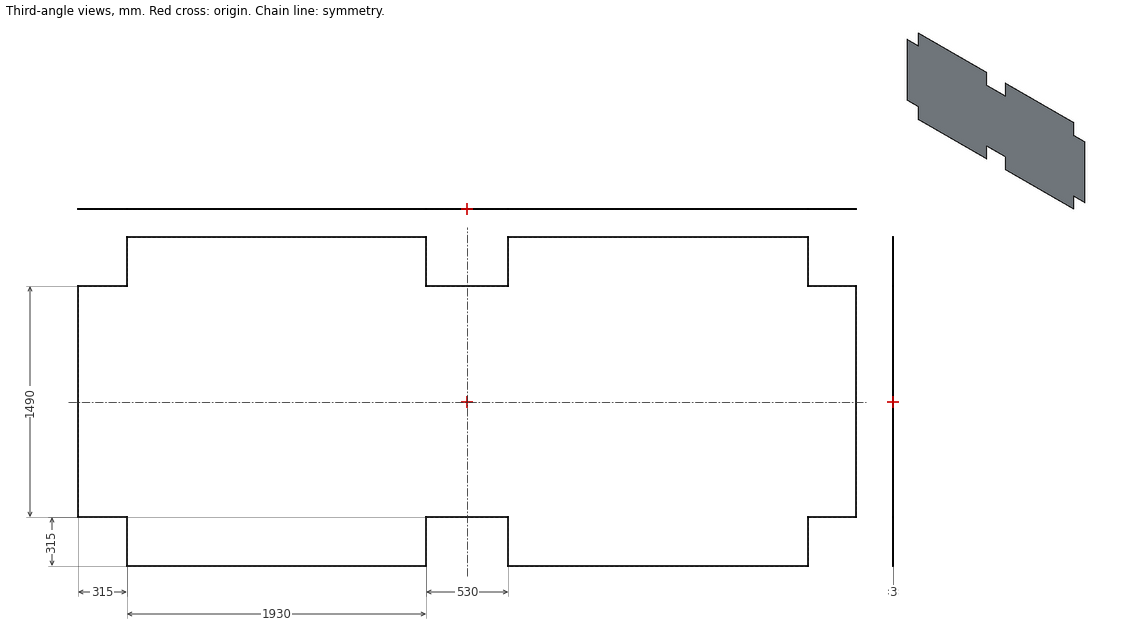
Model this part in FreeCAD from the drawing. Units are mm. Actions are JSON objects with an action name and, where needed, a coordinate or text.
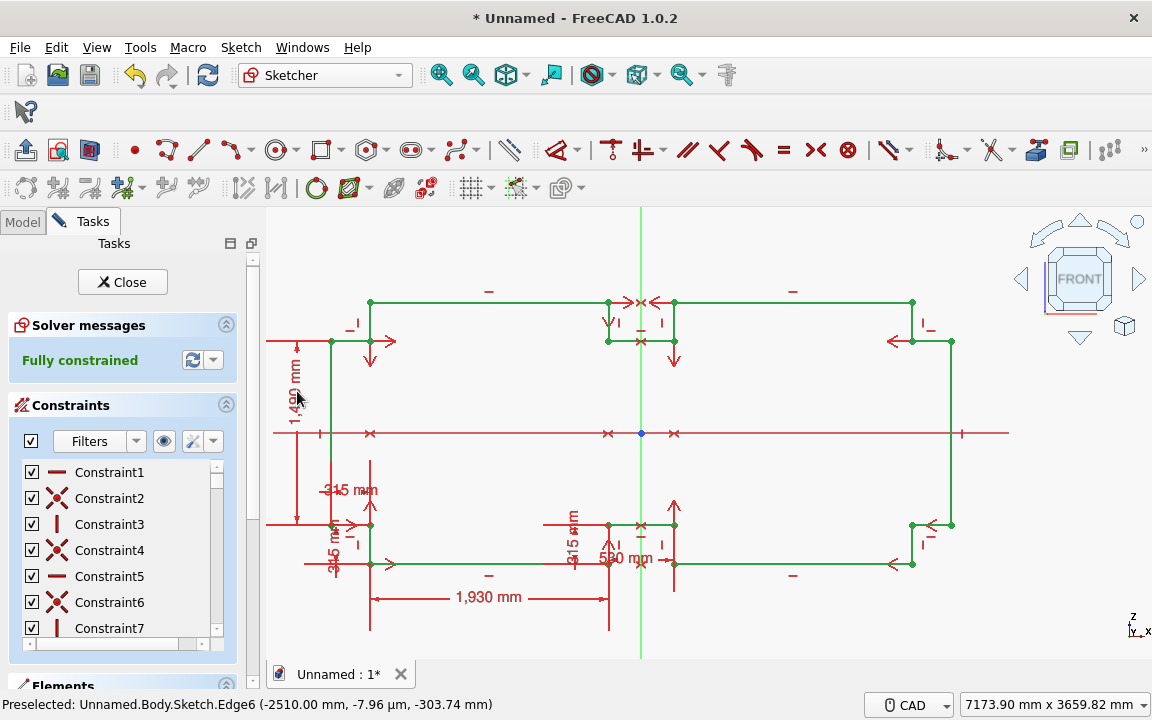
{"action": "left_click", "coordinate": [123, 282]}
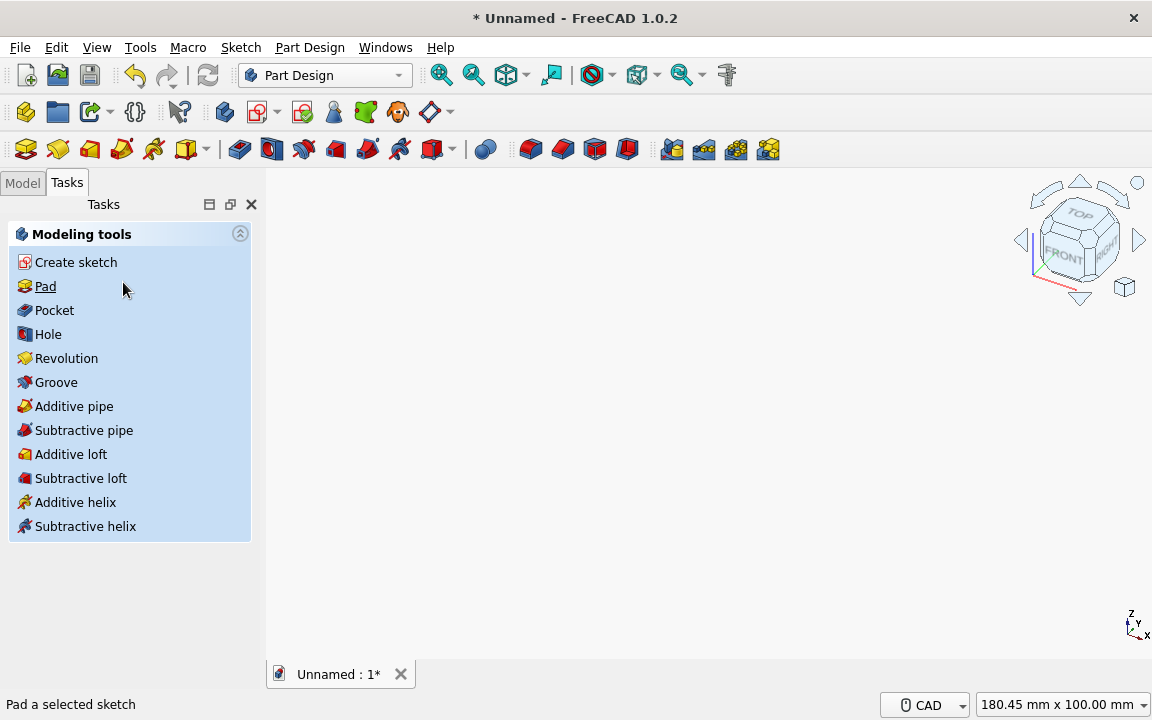
{"action": "left_click", "coordinate": [26, 150]}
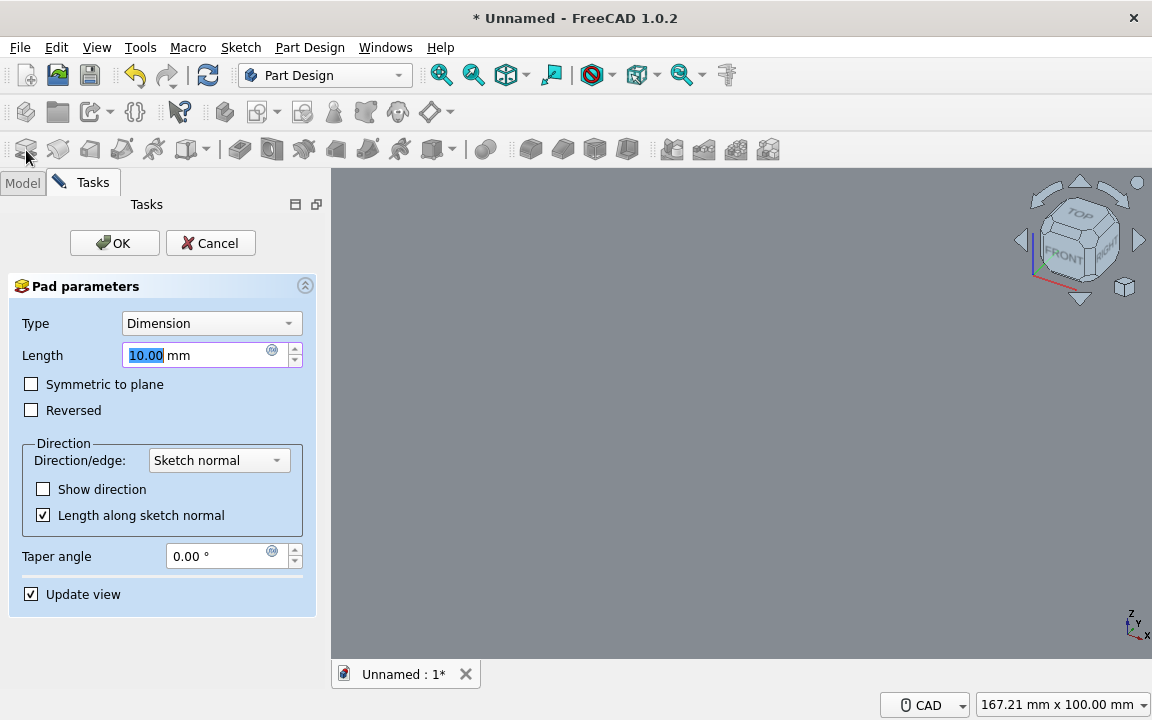
{"action": "type", "text": "3"}
{"action": "key", "text": "Tab"}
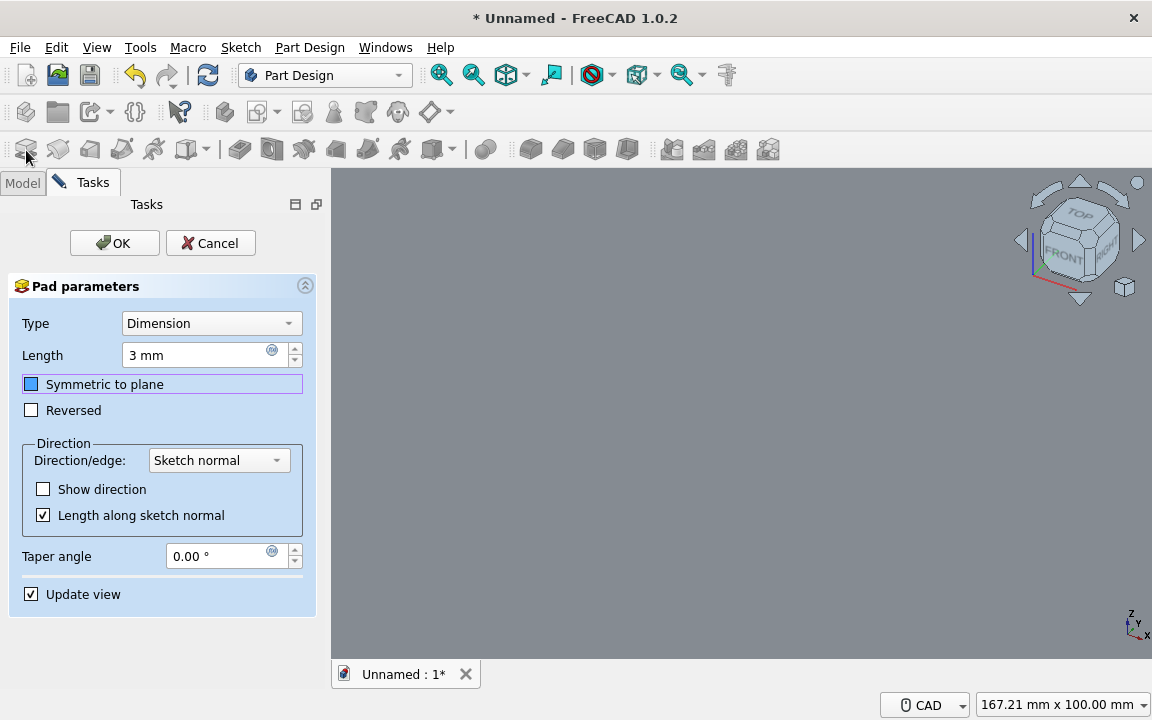
{"action": "left_click", "coordinate": [30, 410]}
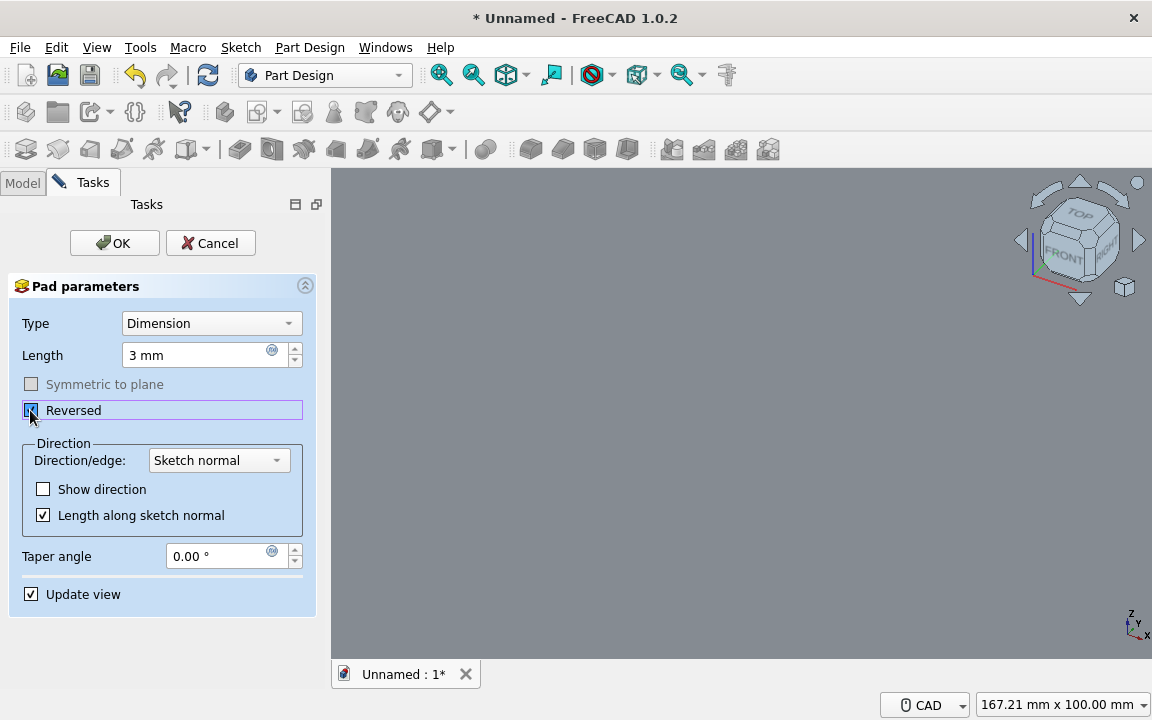
{"action": "left_click", "coordinate": [115, 243]}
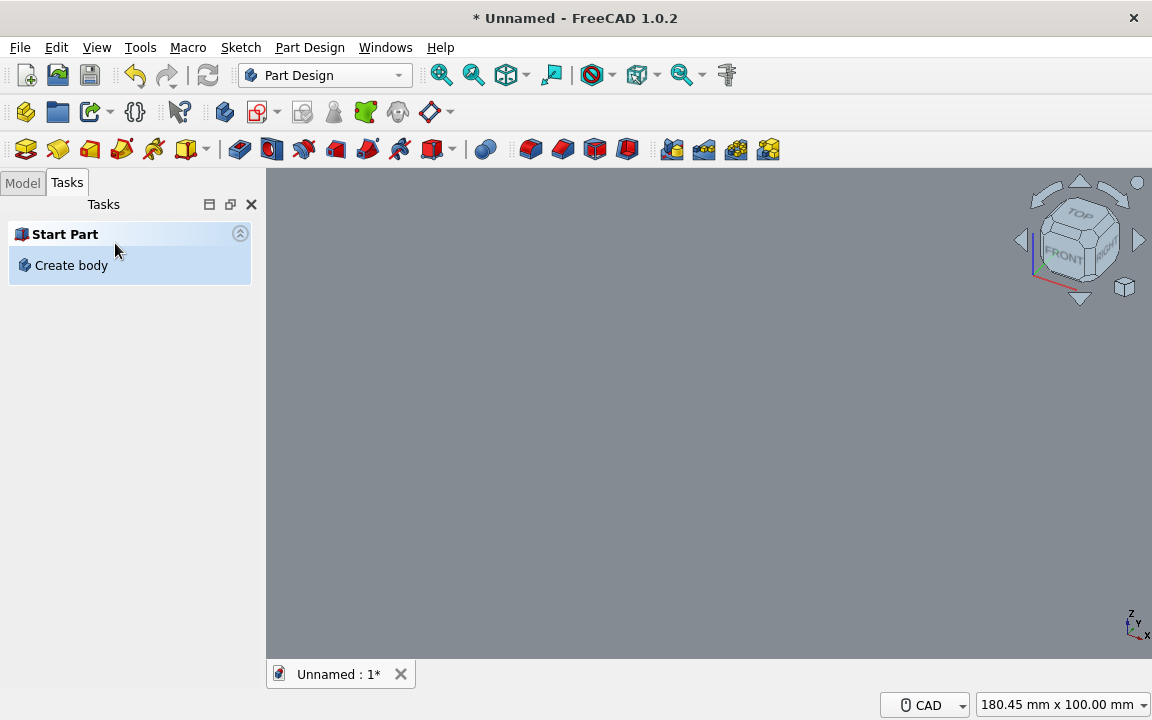
{"action": "key", "text": "0"}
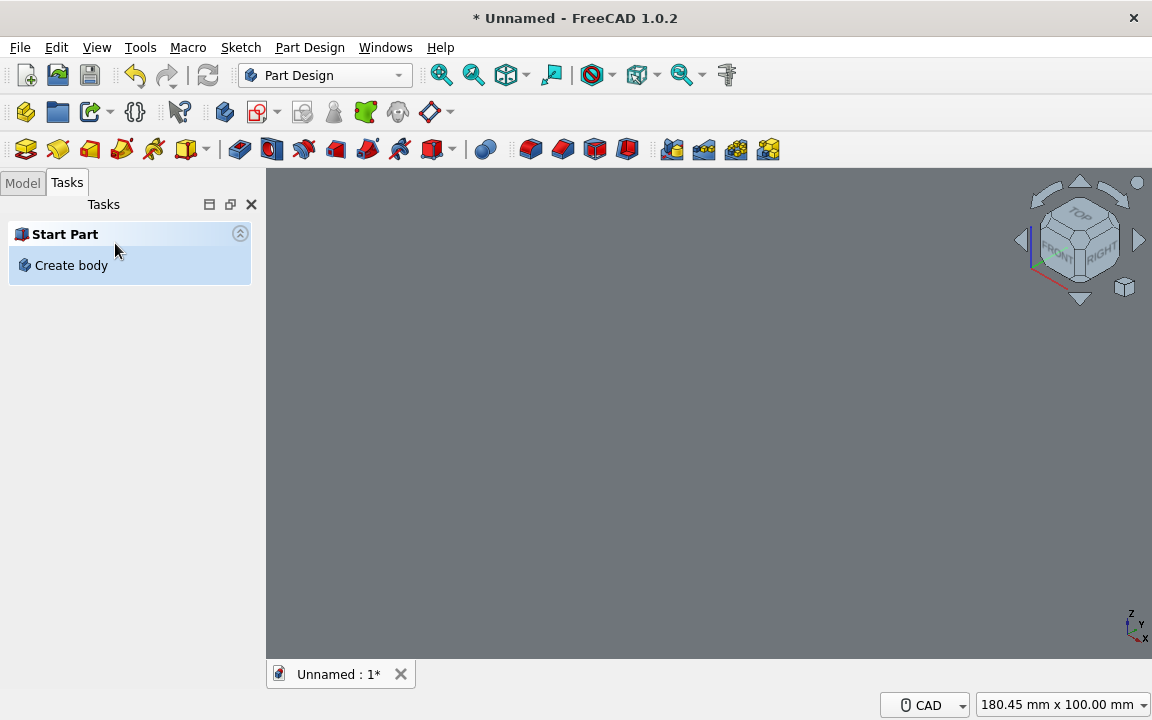
{"action": "left_click", "coordinate": [442, 76]}